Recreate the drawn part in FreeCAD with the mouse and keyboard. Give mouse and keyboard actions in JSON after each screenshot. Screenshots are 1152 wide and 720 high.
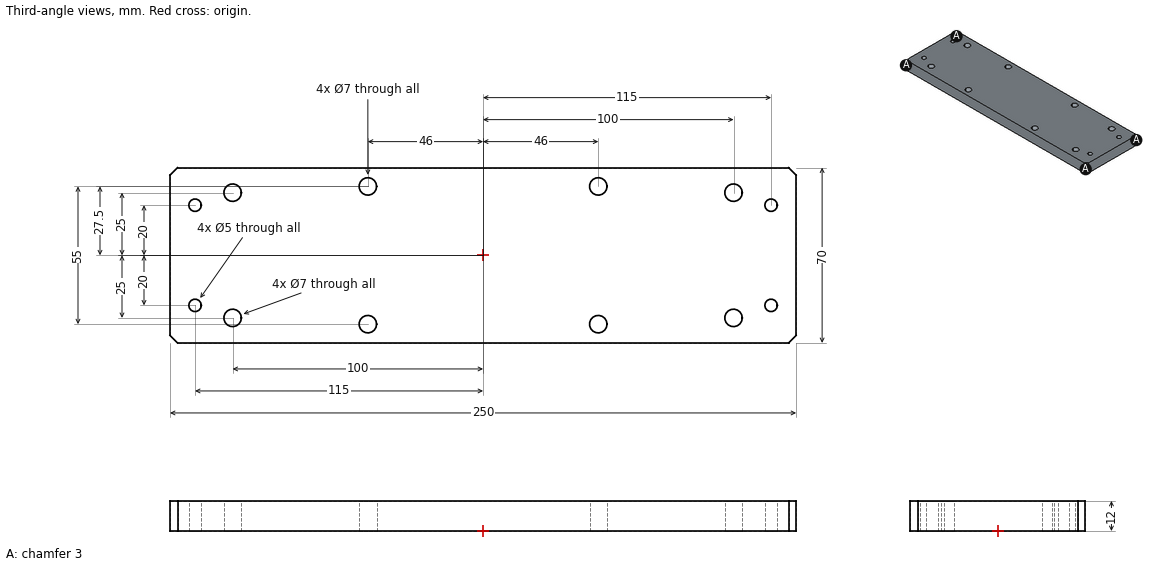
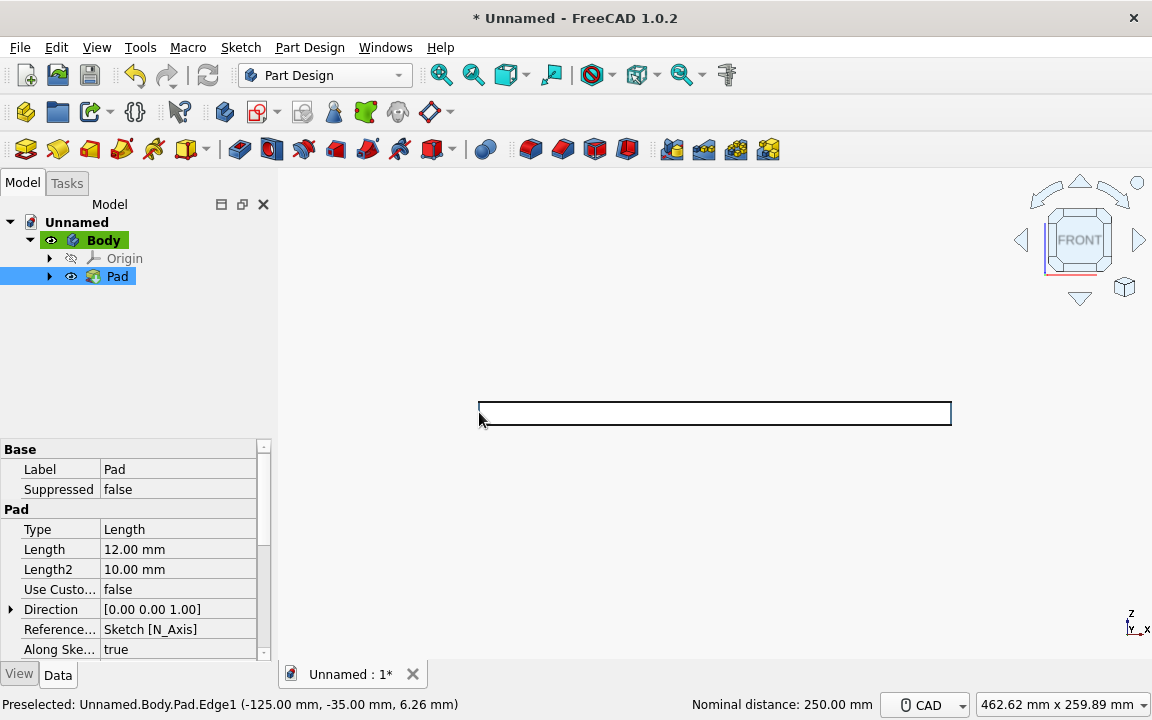
{"action": "key", "text": "3"}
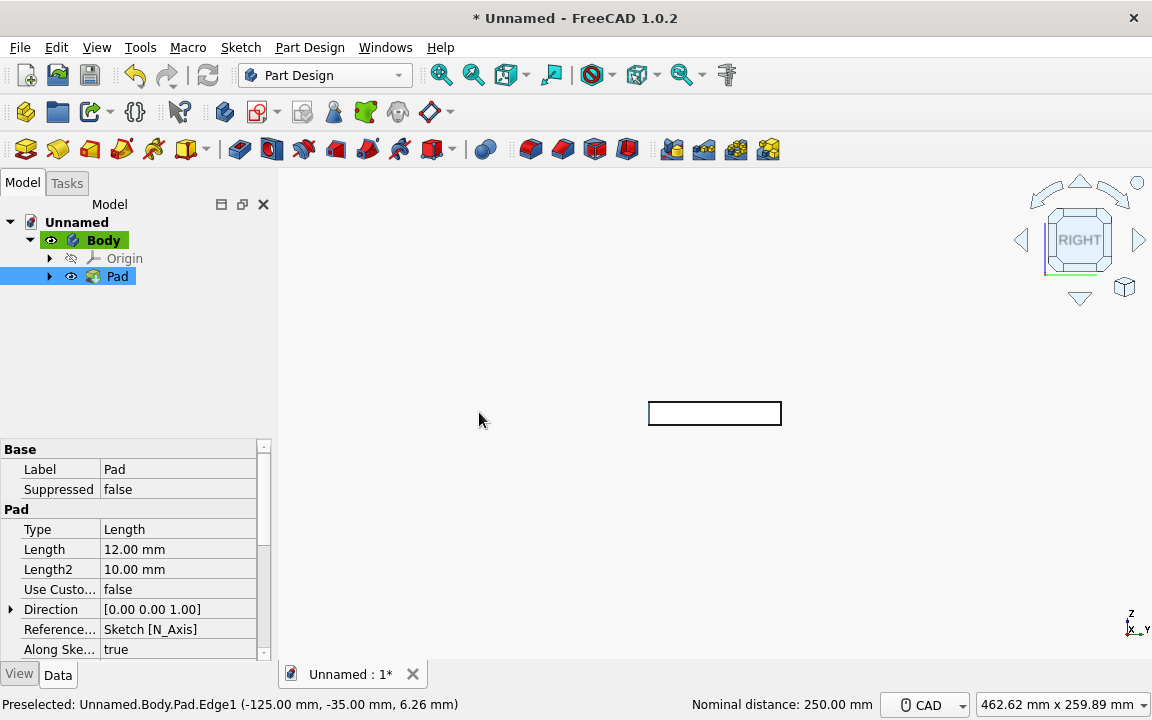
{"action": "left_click", "coordinate": [442, 76]}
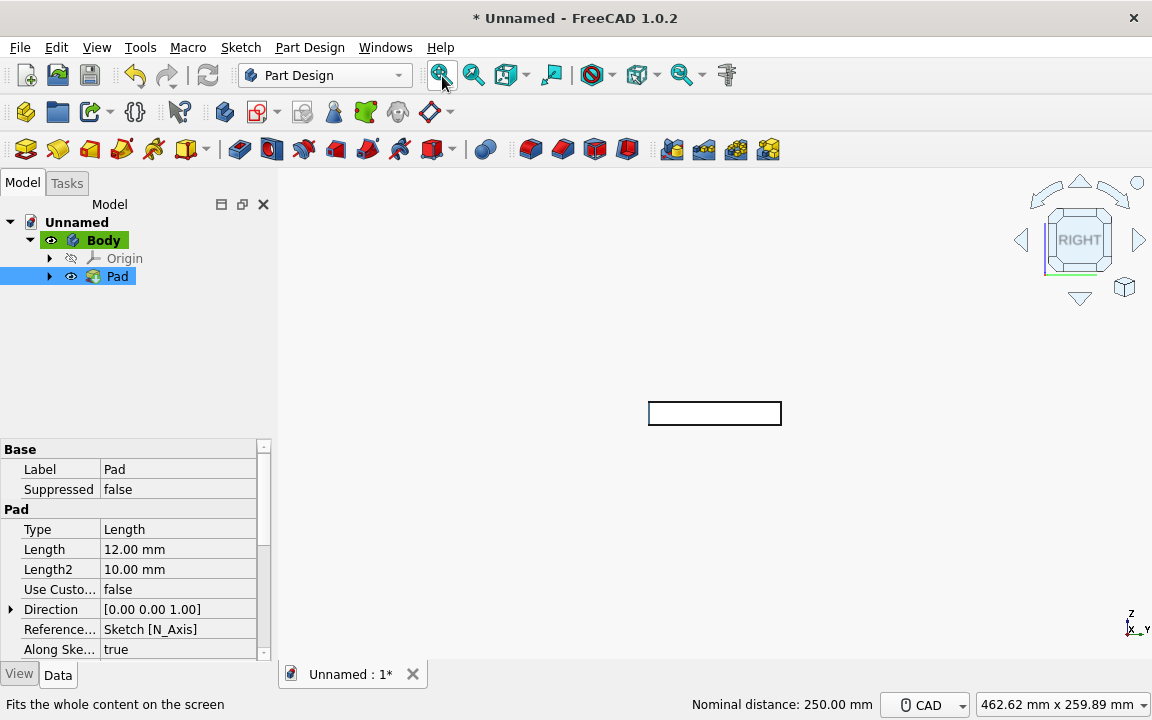
{"action": "left_click", "coordinate": [781, 412], "text": "ctrl"}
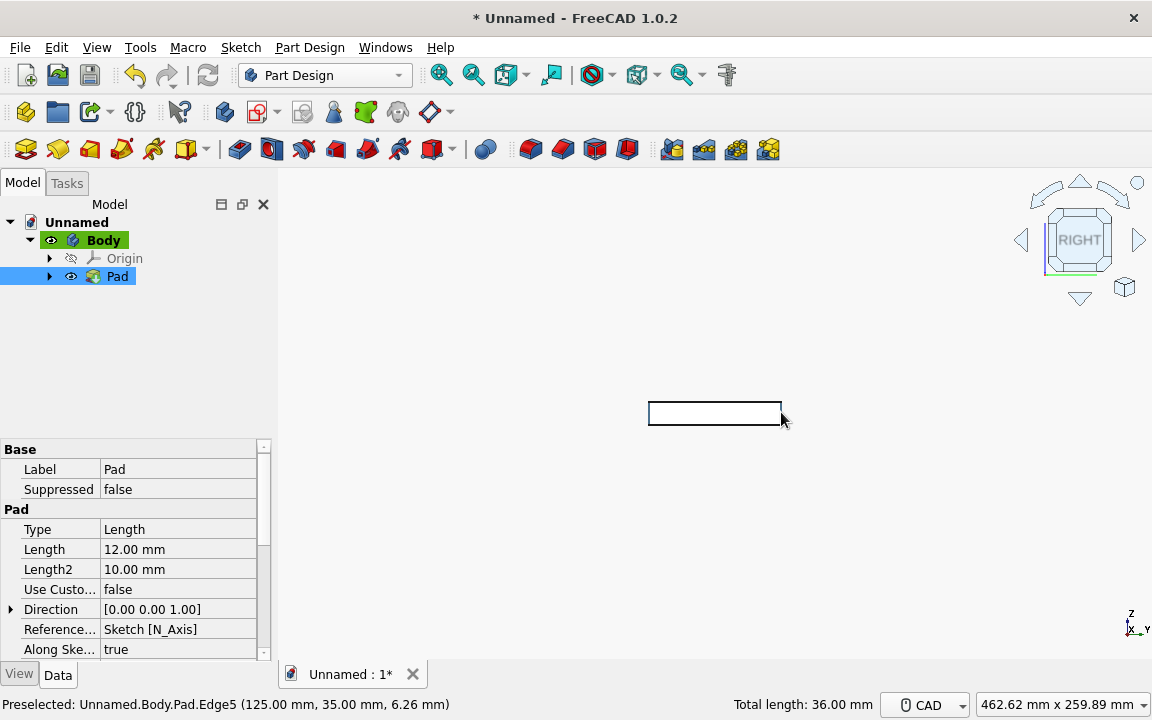
{"action": "key", "text": "5"}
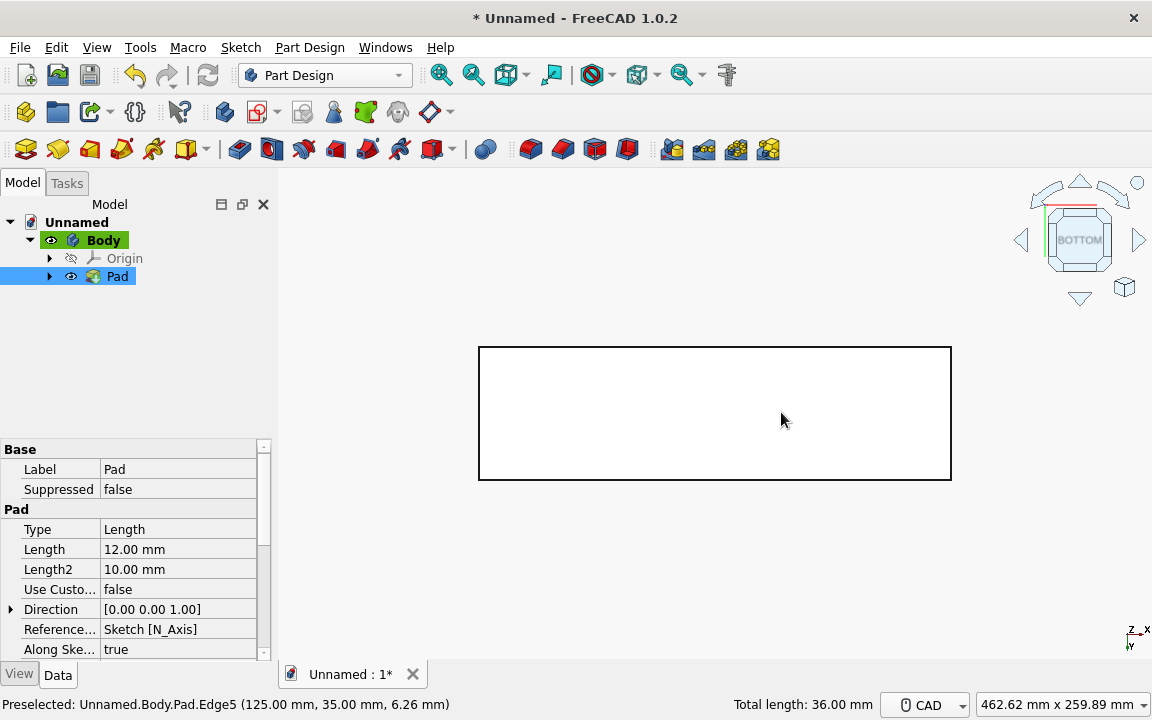
{"action": "key", "text": "4"}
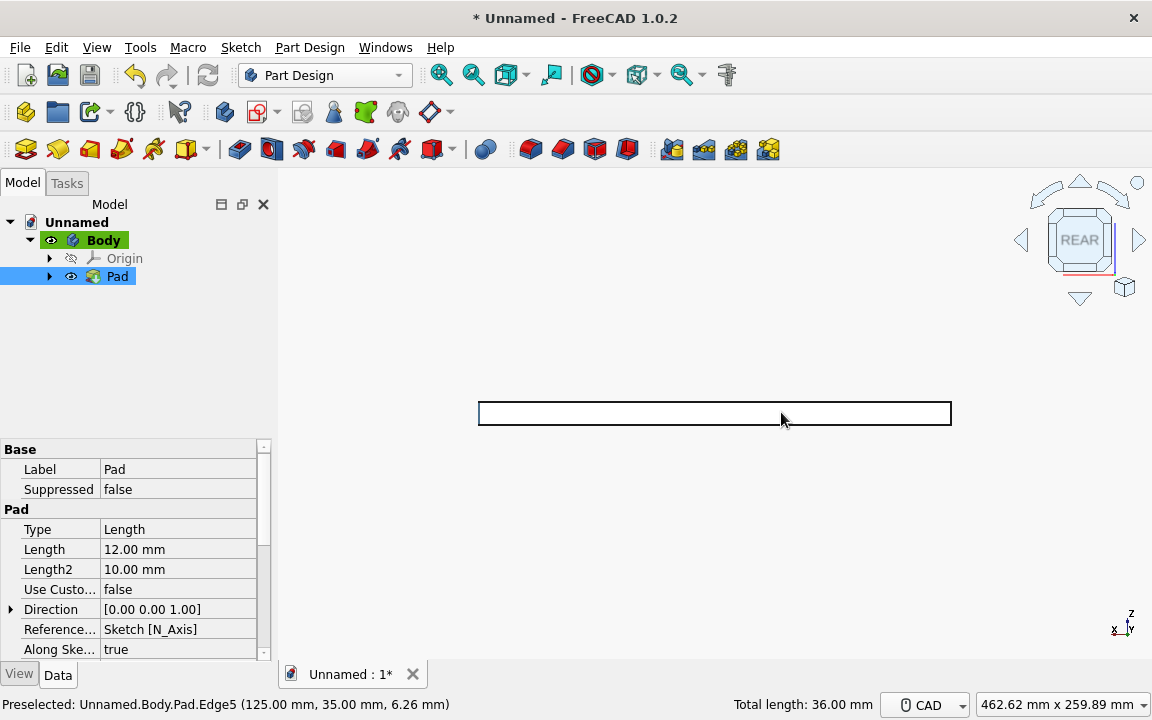
{"action": "left_click", "coordinate": [951, 412], "text": "ctrl"}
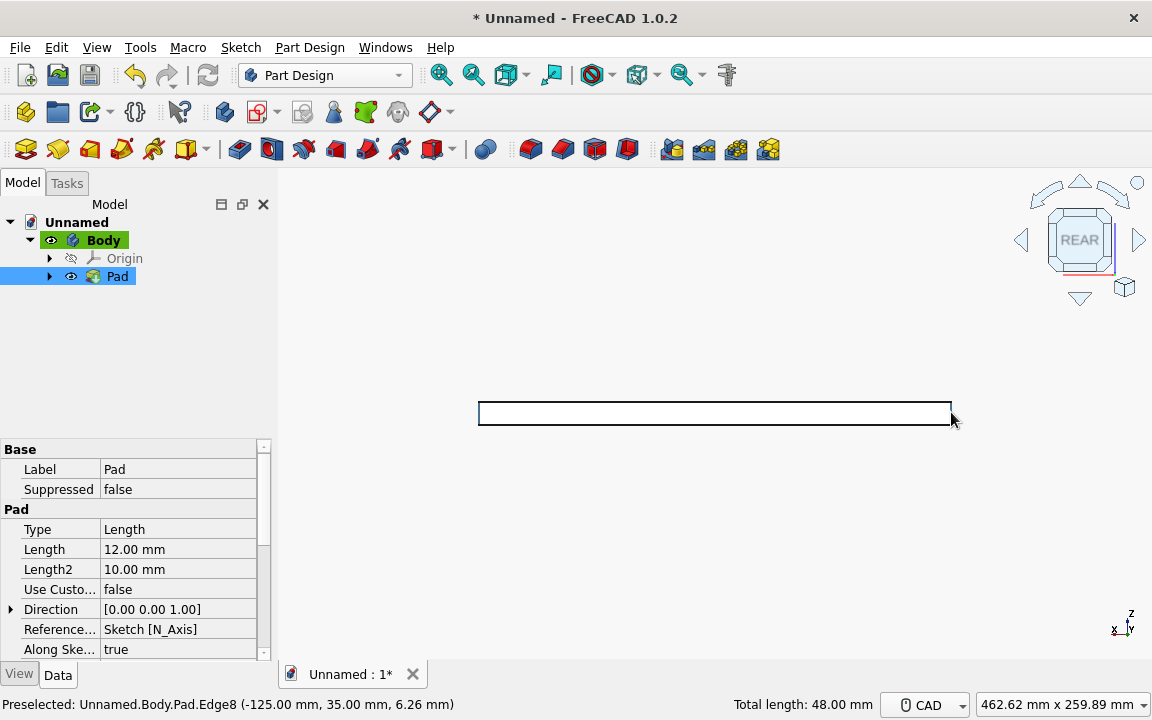
{"action": "left_click", "coordinate": [564, 150]}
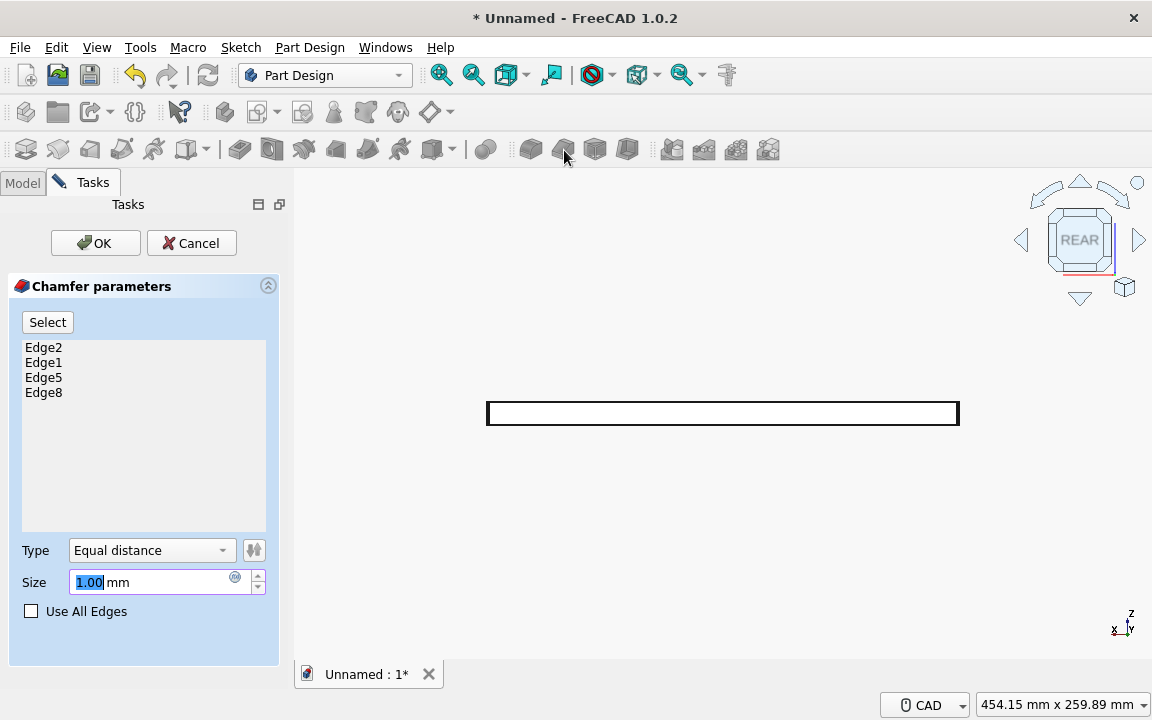
{"action": "type", "text": "3"}
{"action": "key", "text": "Tab"}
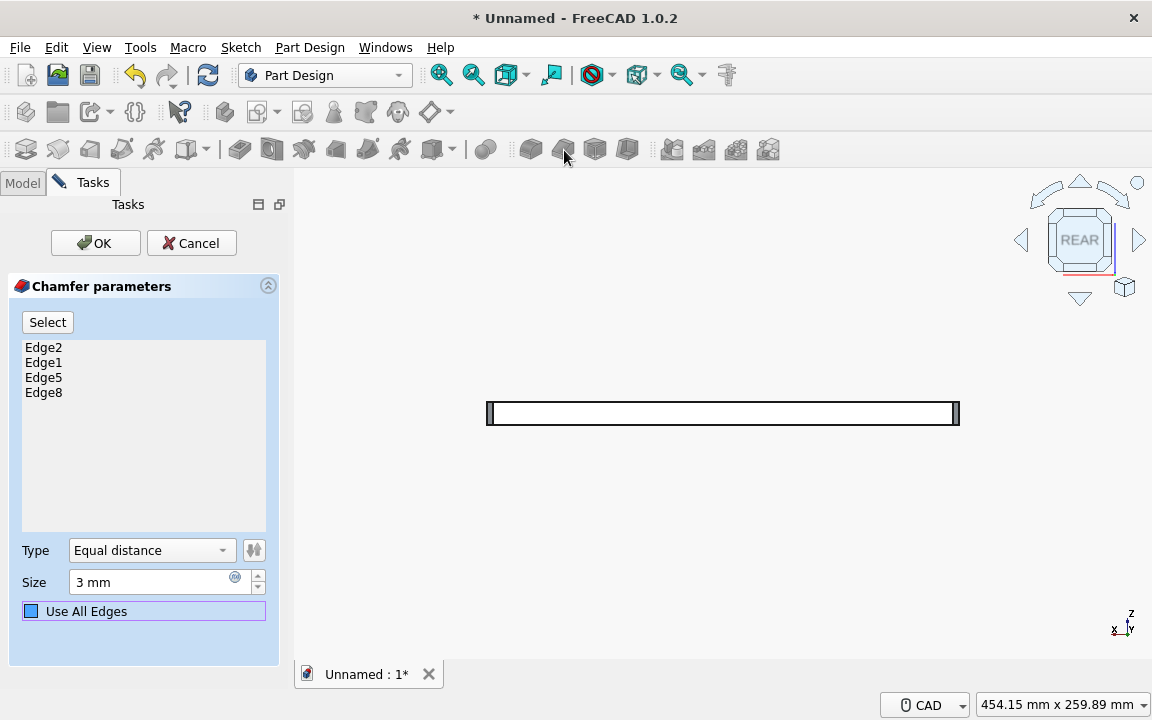
{"action": "left_click", "coordinate": [96, 243]}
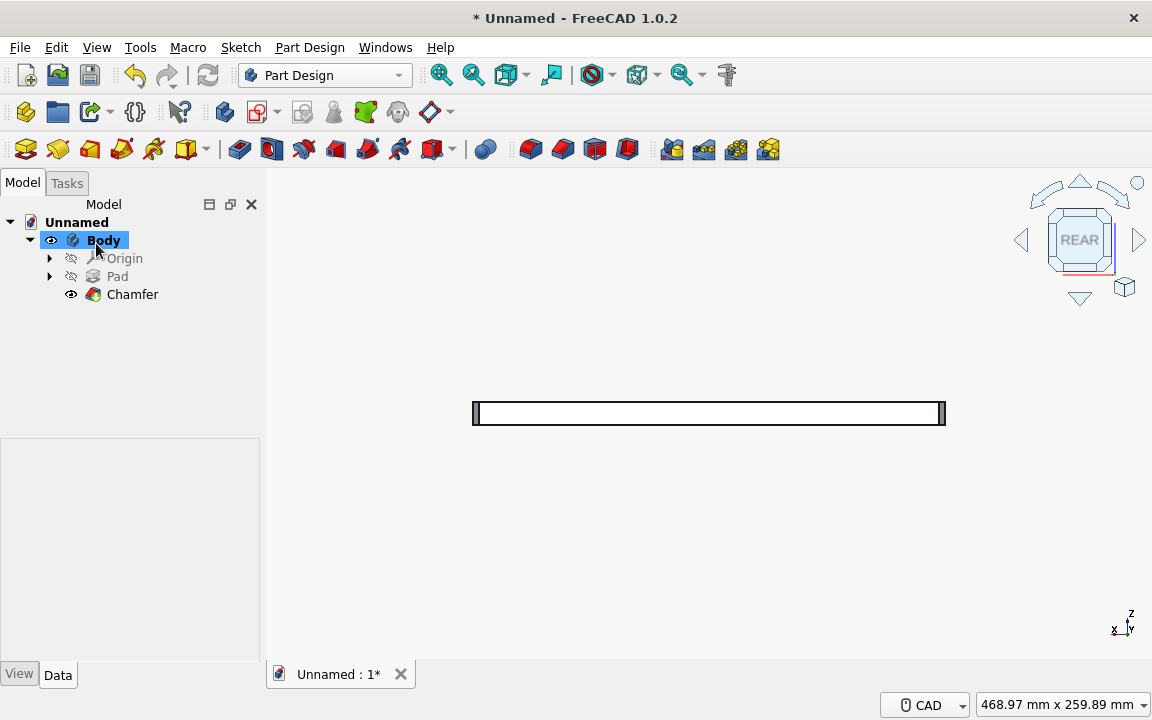
{"action": "key", "text": "5"}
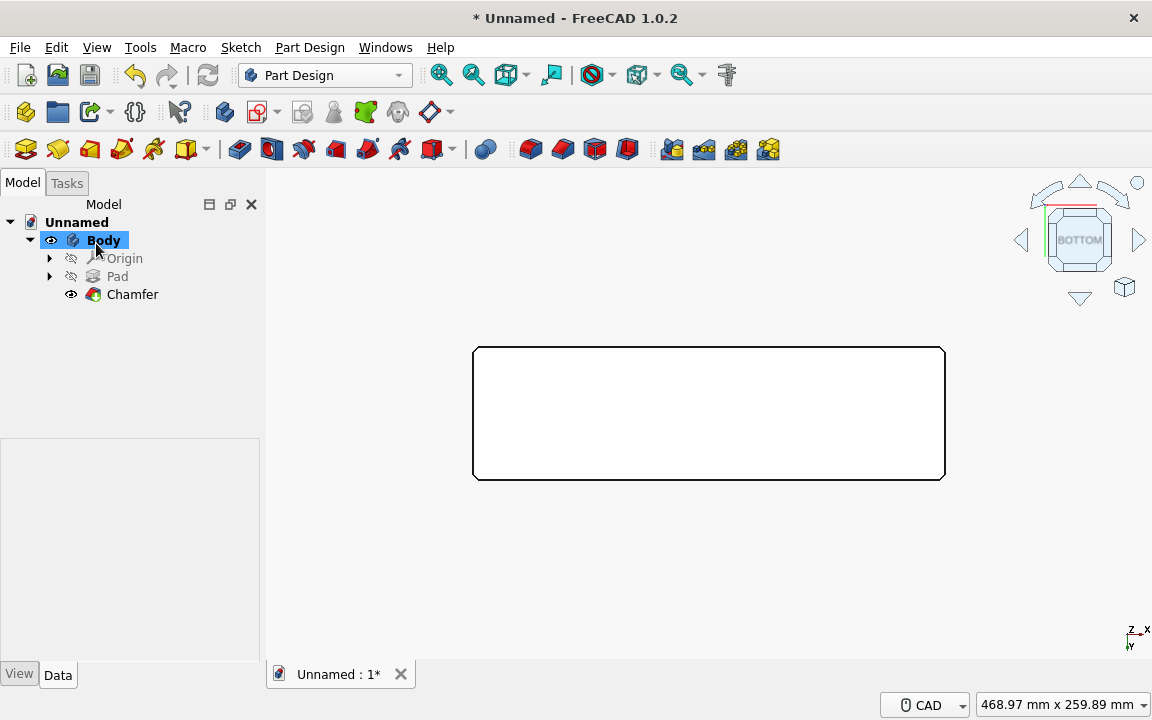
{"action": "left_click", "coordinate": [844, 412]}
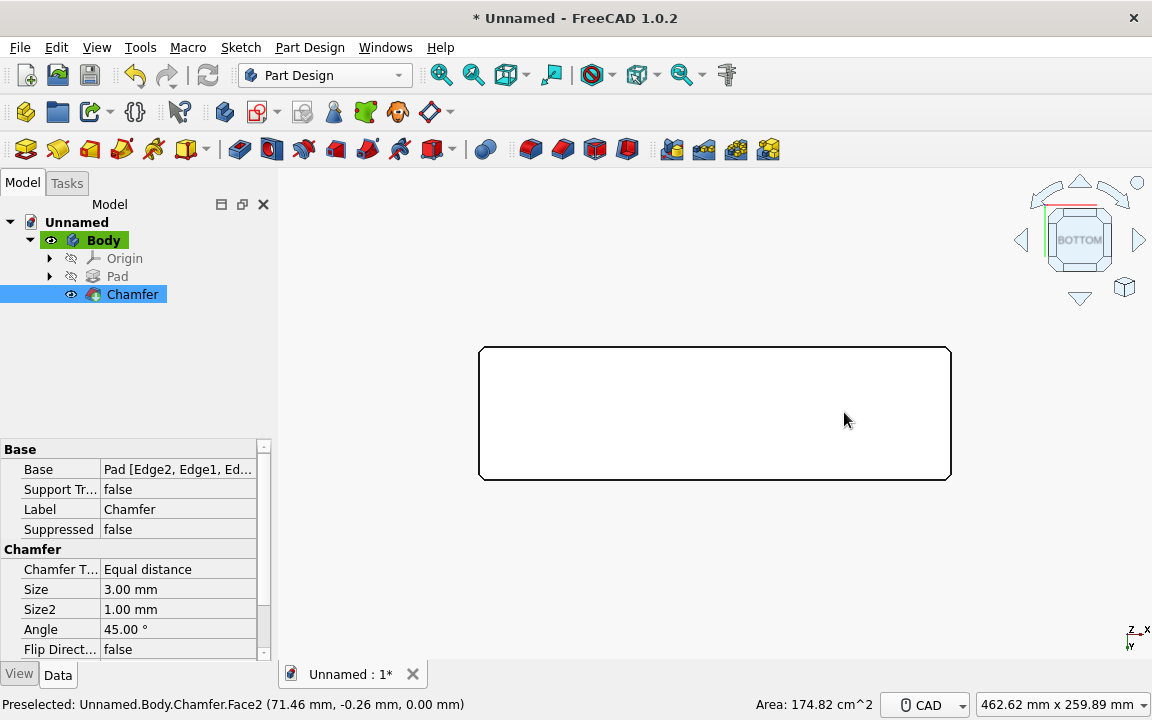
{"action": "left_click", "coordinate": [258, 112]}